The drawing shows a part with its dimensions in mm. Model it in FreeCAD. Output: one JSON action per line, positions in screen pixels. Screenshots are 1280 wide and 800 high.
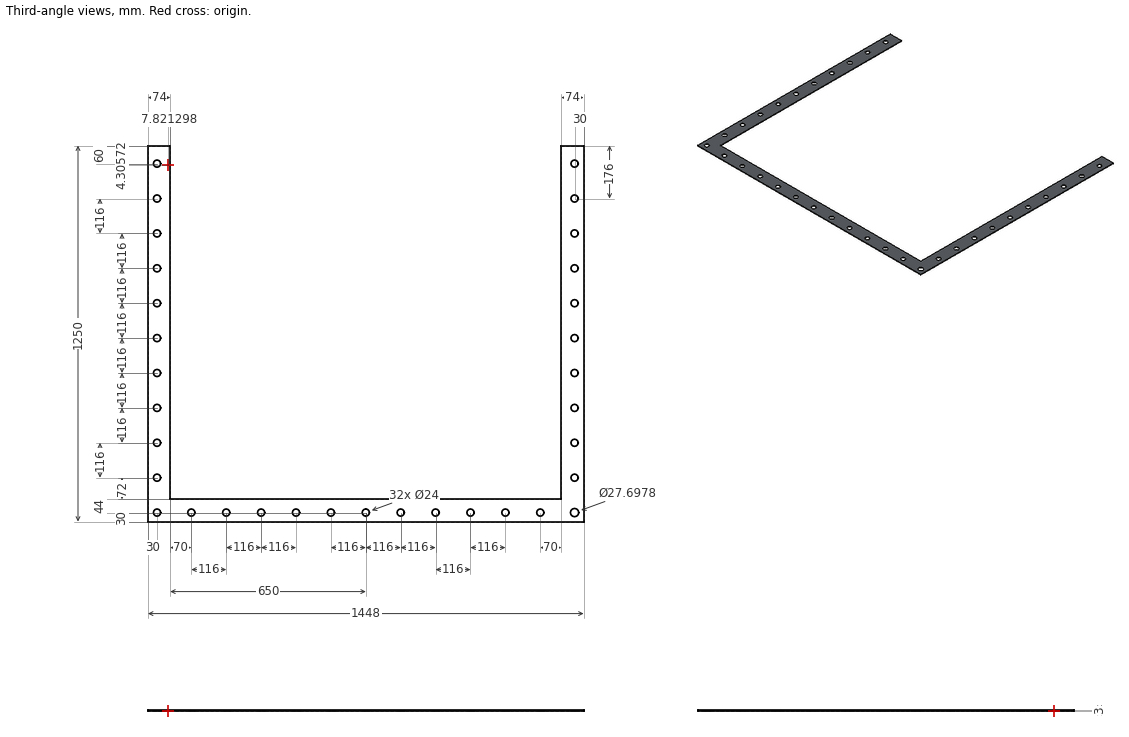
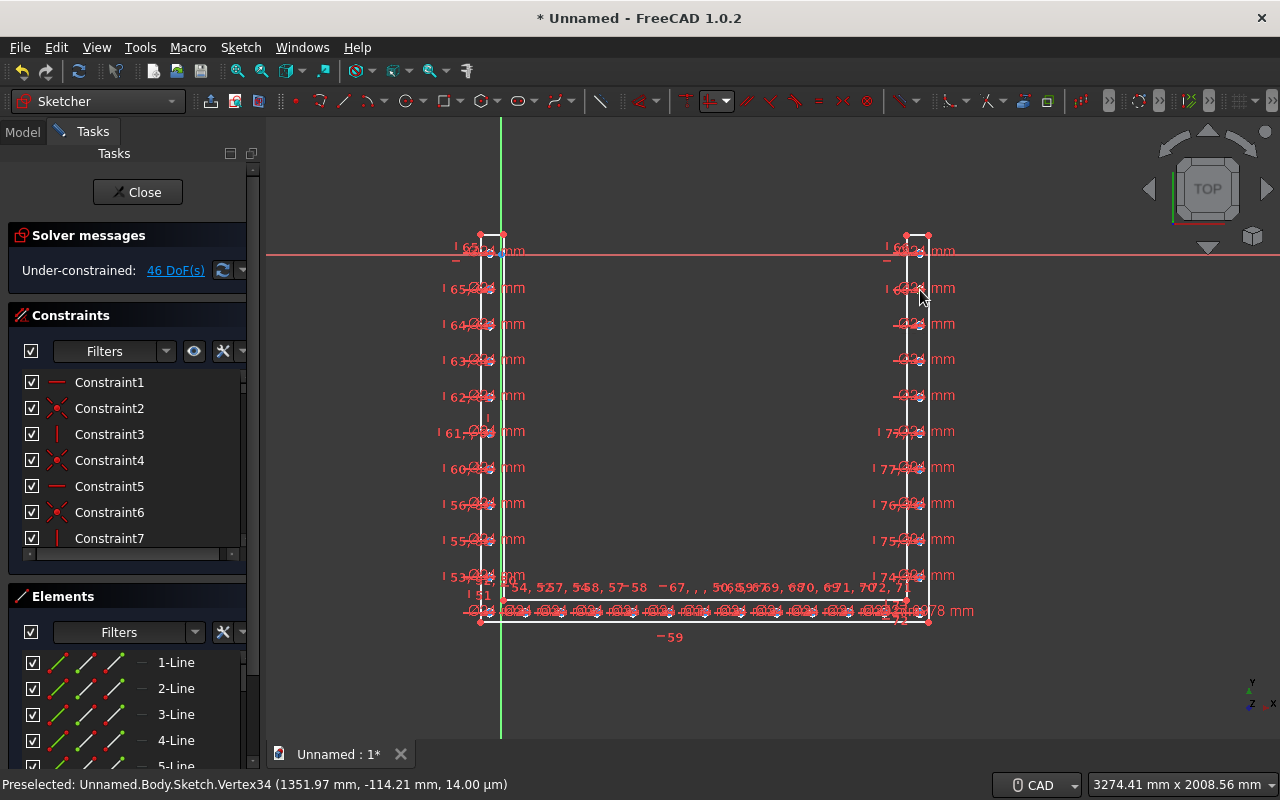
{"action": "left_click", "coordinate": [920, 433]}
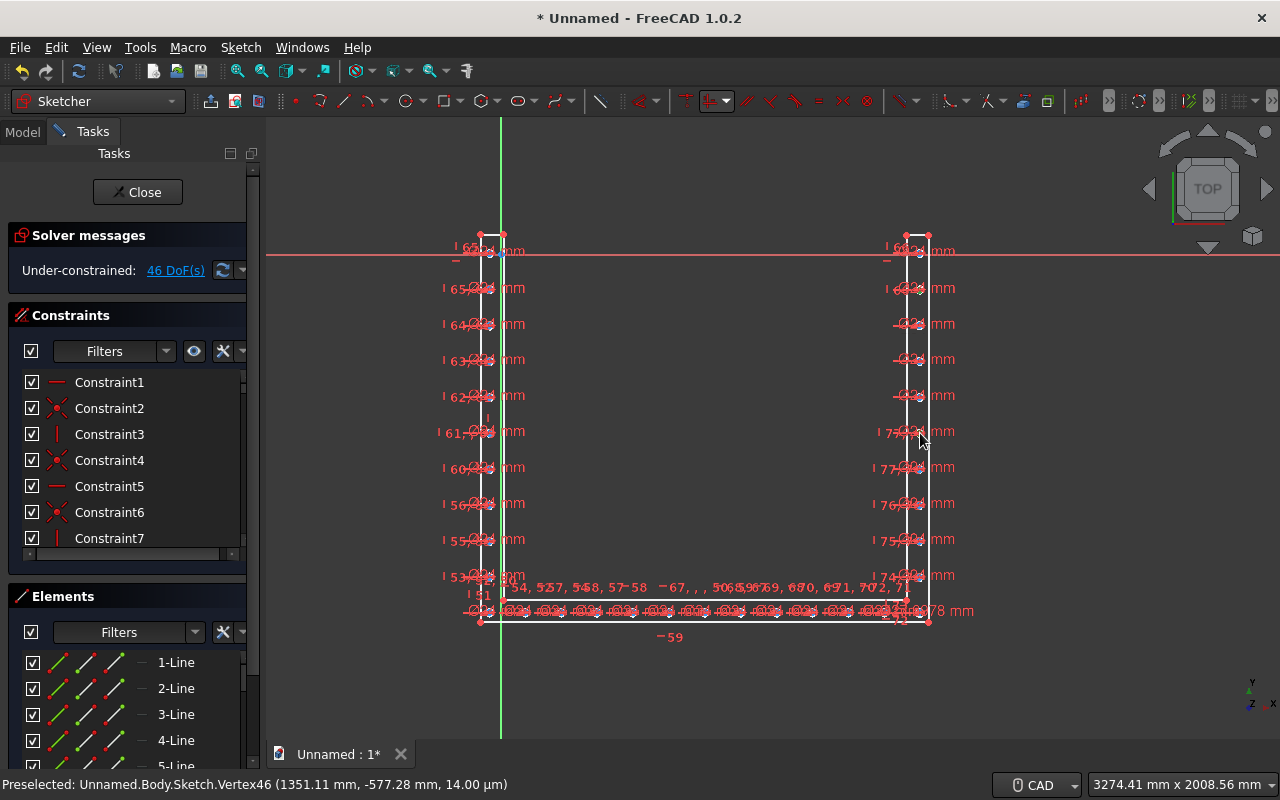
{"action": "key", "text": "v"}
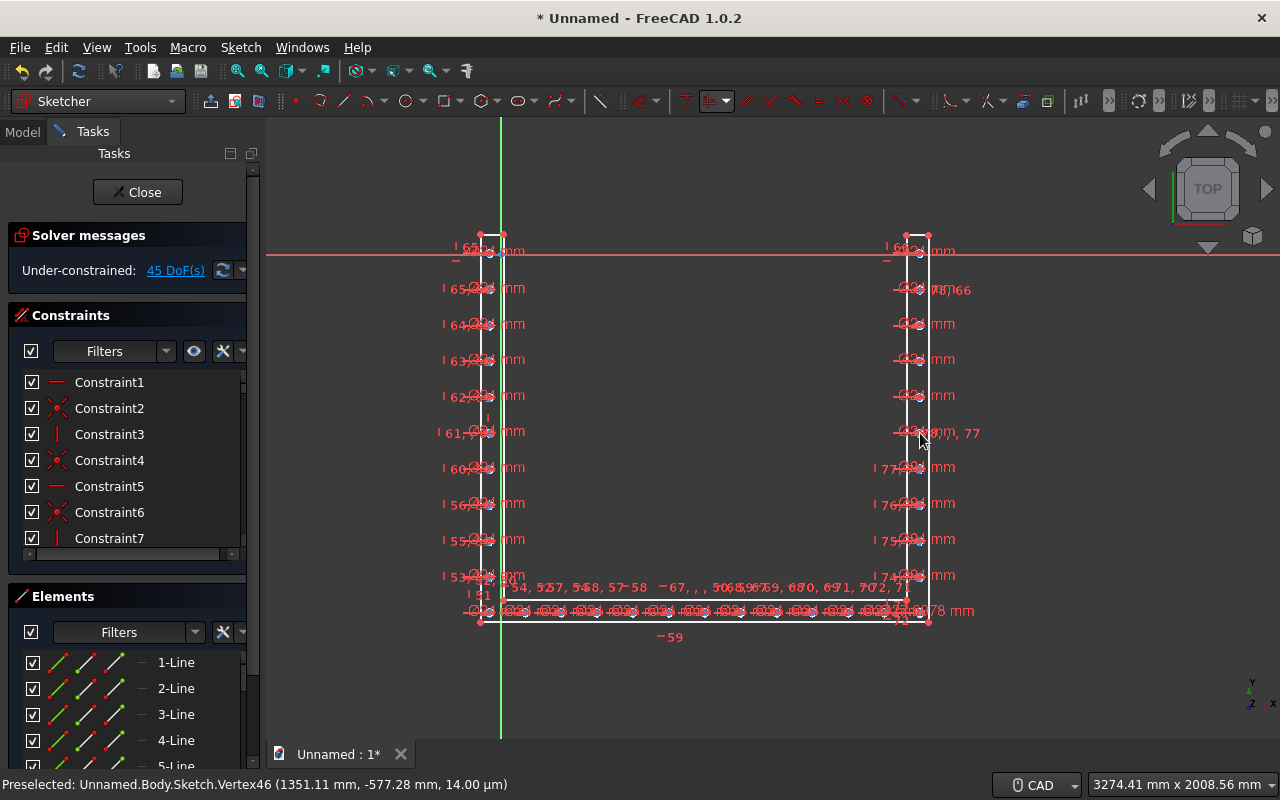
{"action": "scroll", "coordinate": [920, 433], "scroll_direction": "up", "scroll_amount": 4}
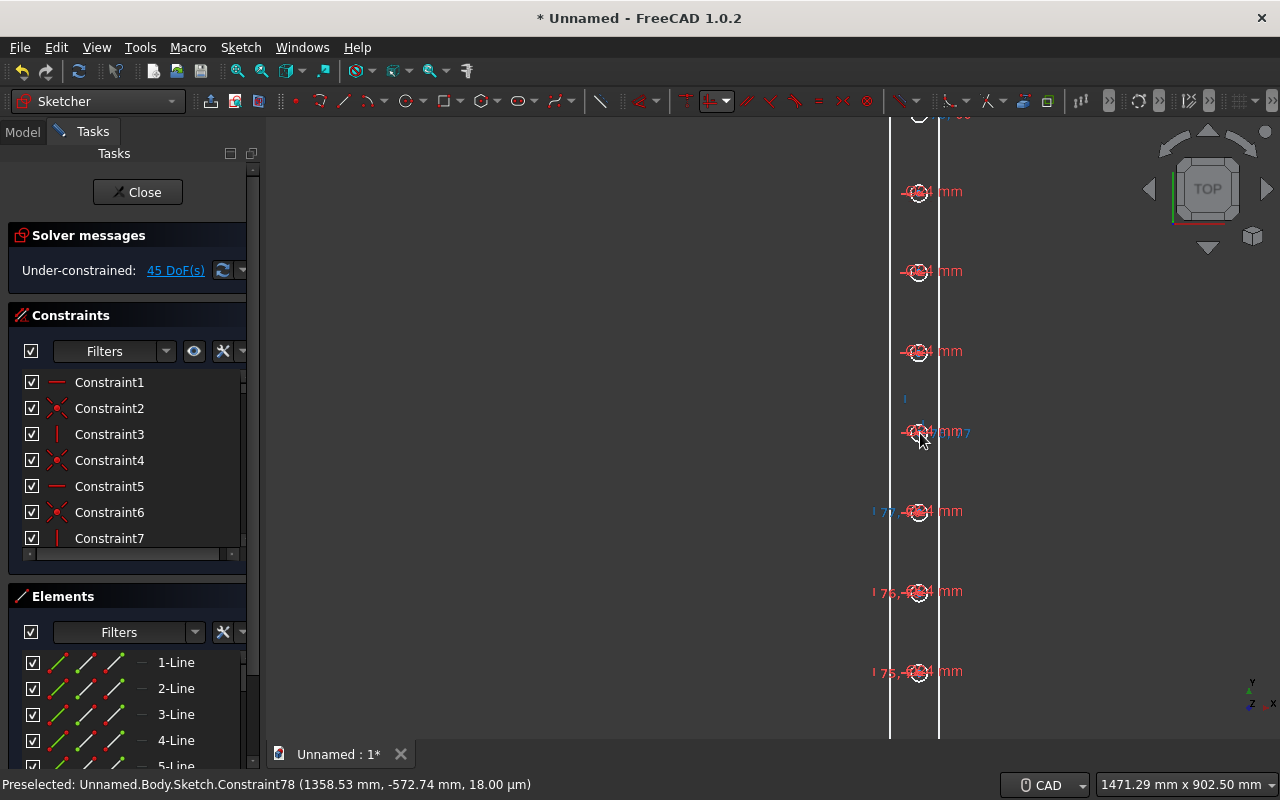
{"action": "left_click", "coordinate": [917, 435]}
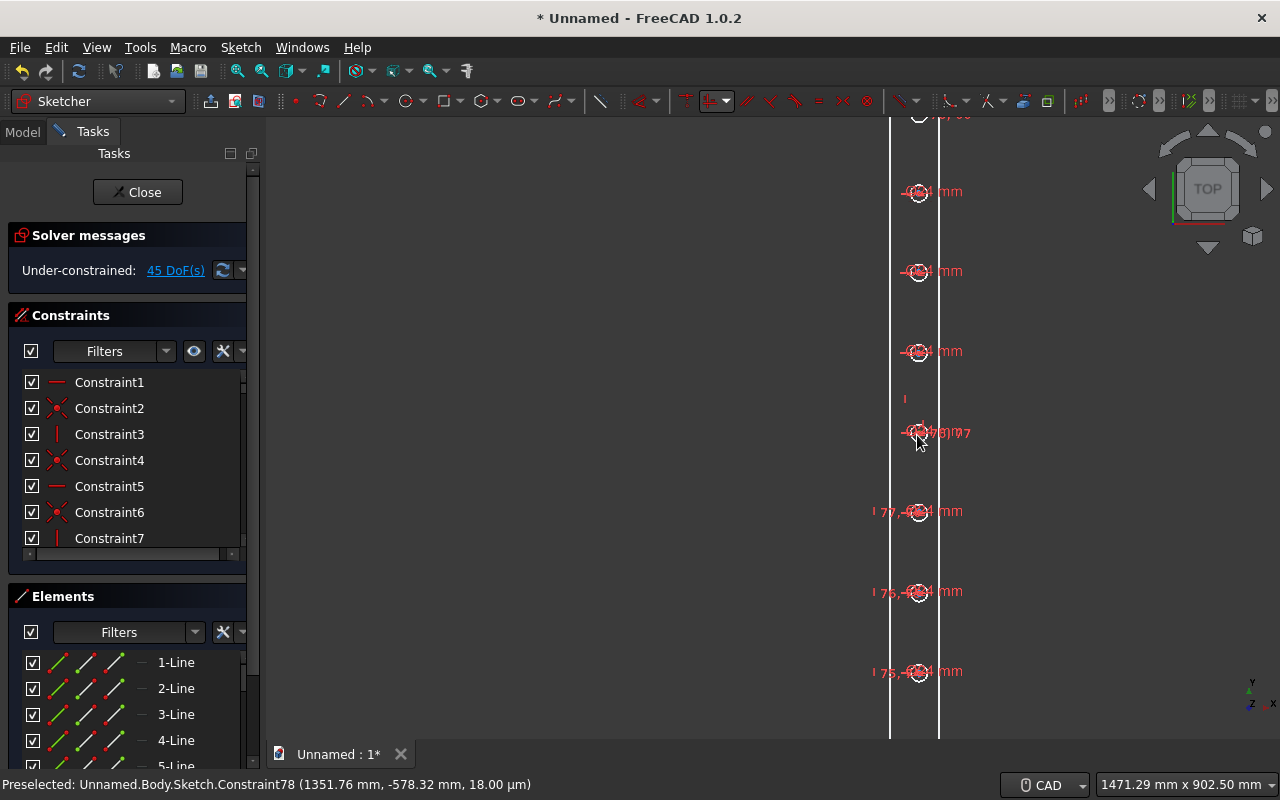
{"action": "left_click", "coordinate": [919, 353]}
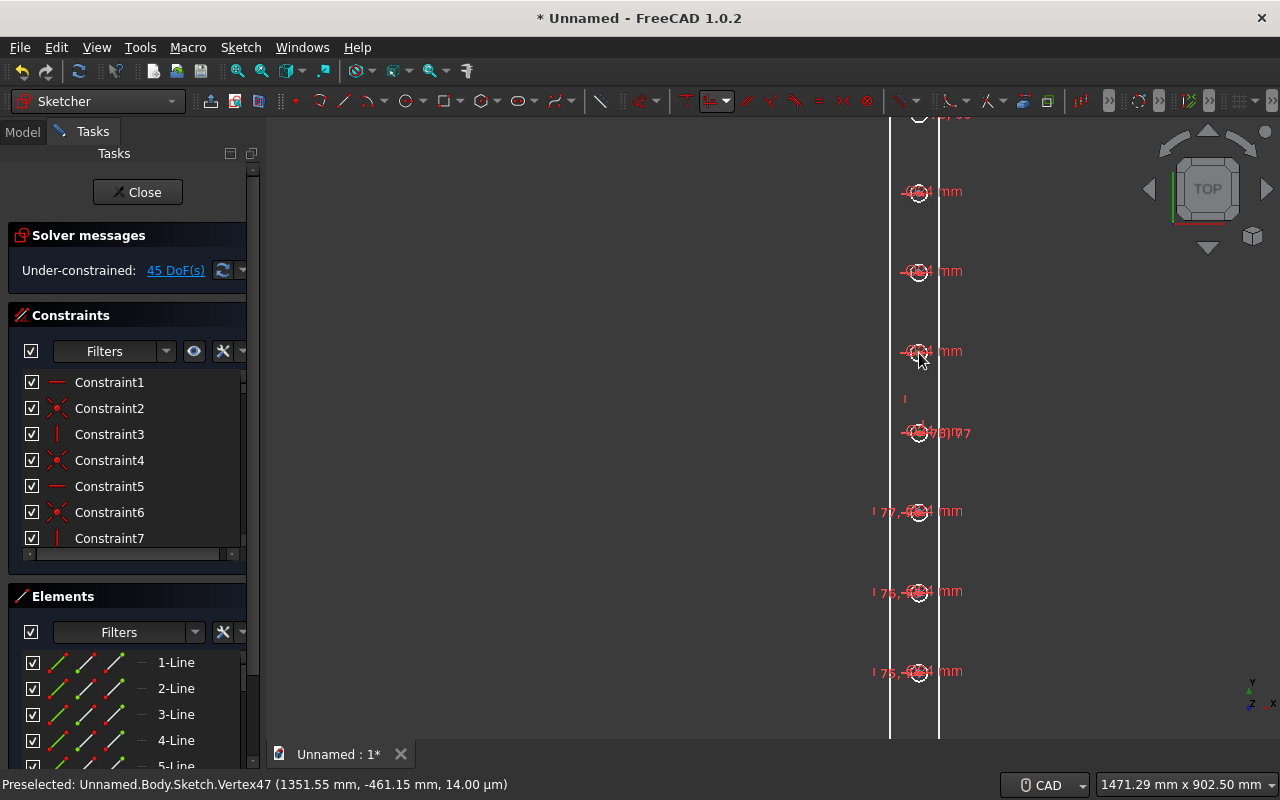
{"action": "left_click", "coordinate": [728, 102]}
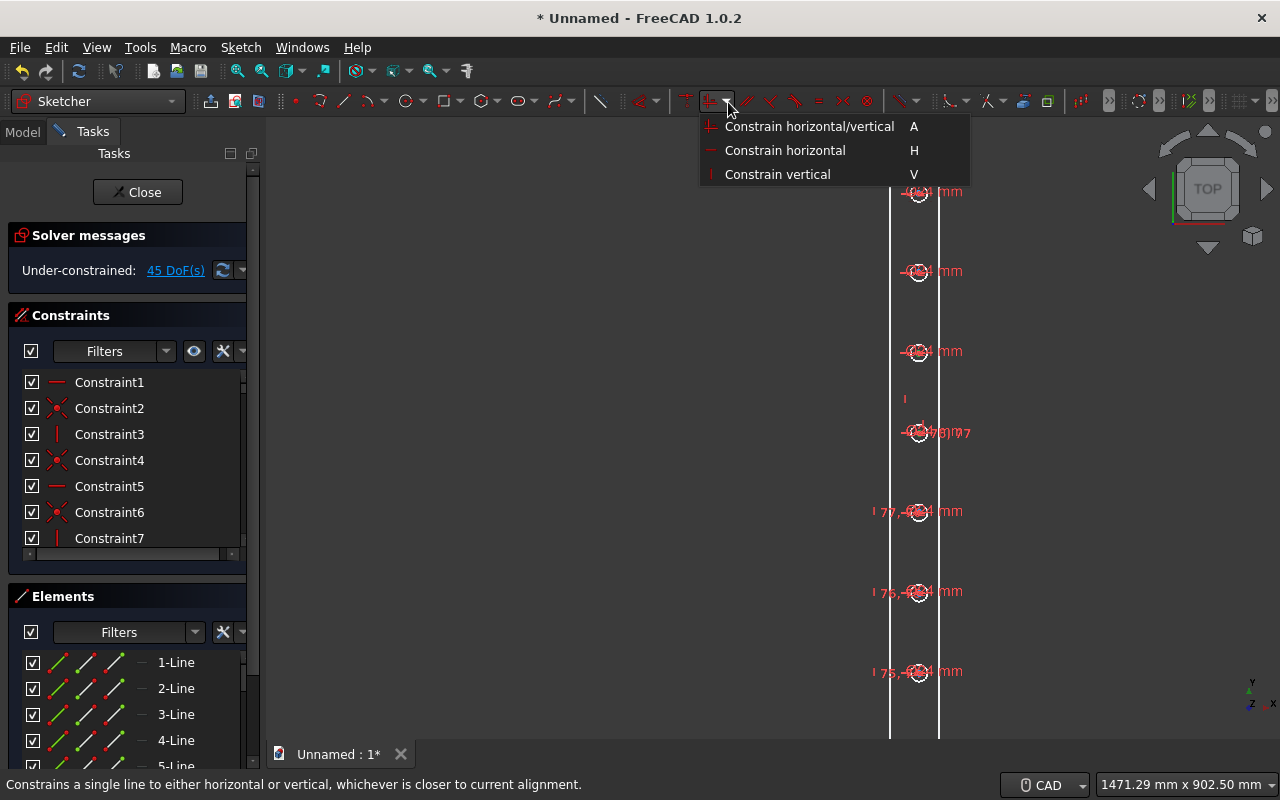
{"action": "left_click", "coordinate": [835, 174]}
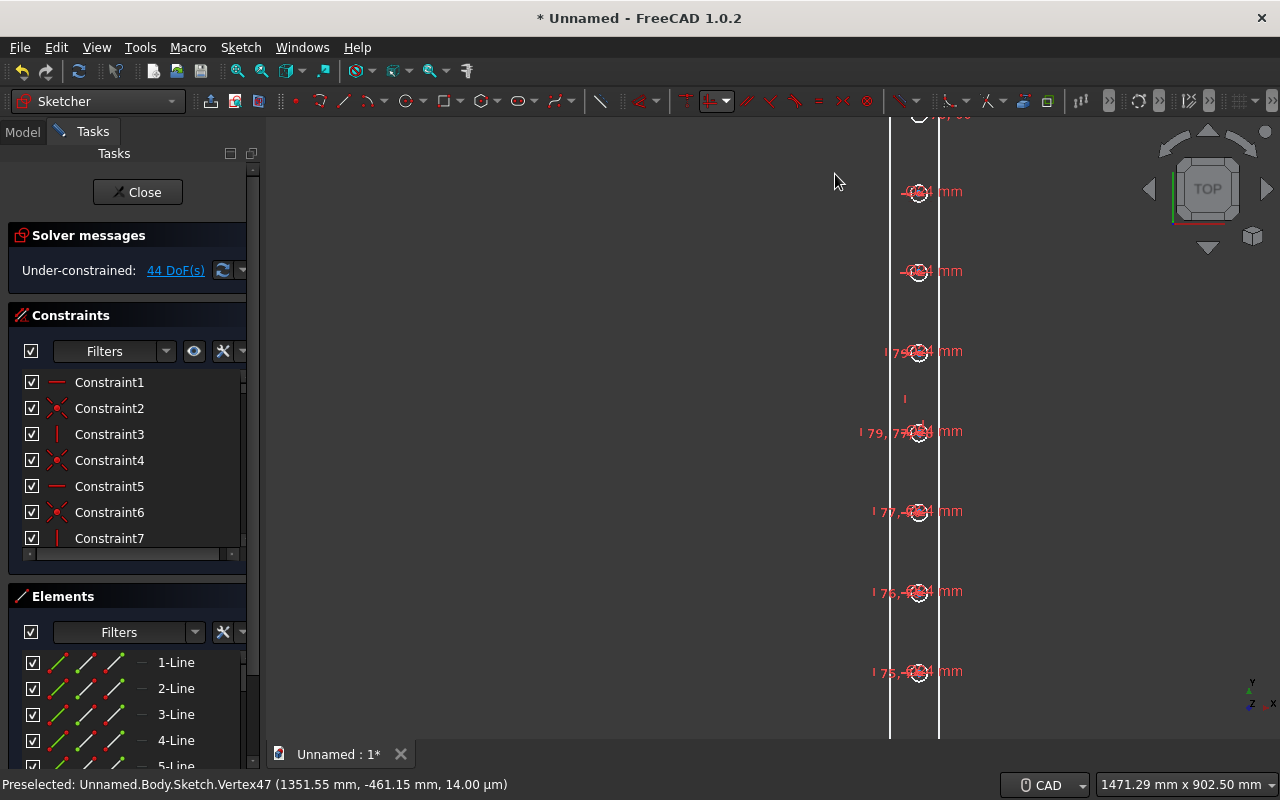
{"action": "left_click", "coordinate": [919, 353]}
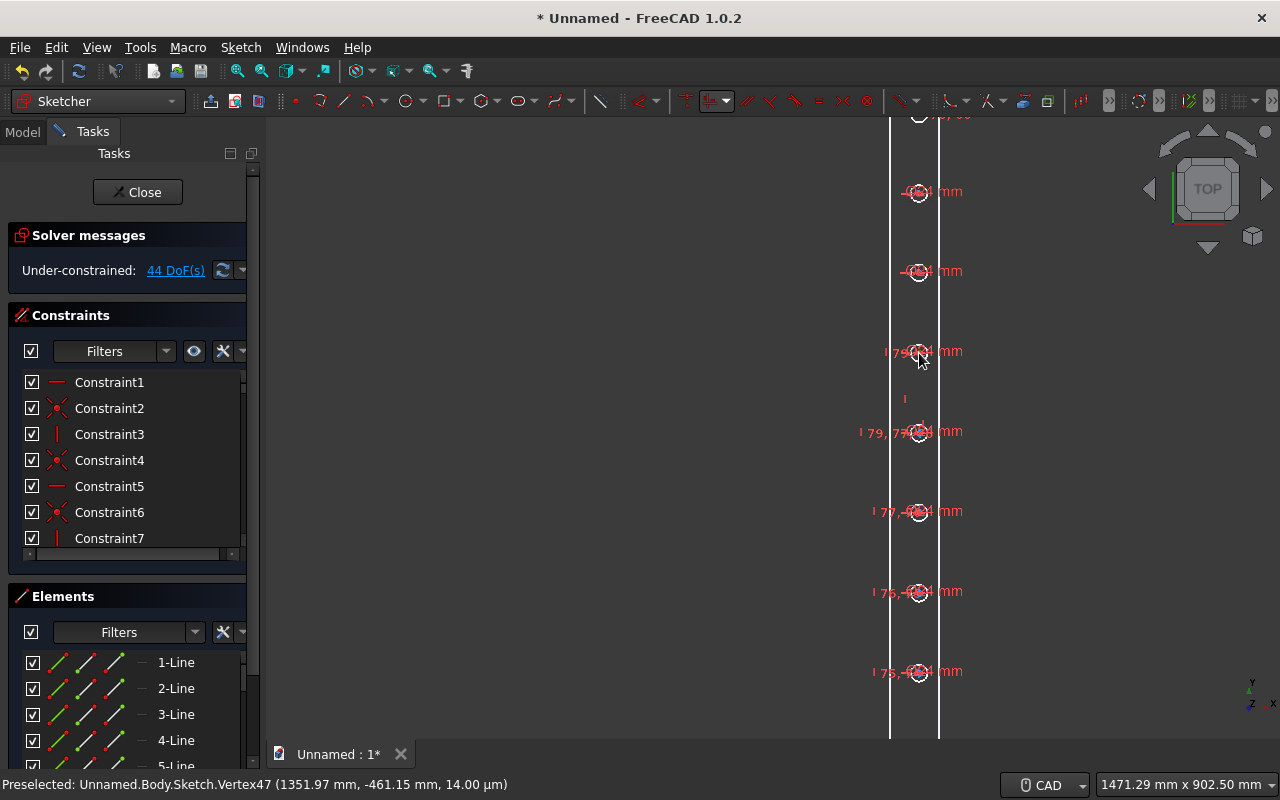
{"action": "left_click", "coordinate": [919, 273]}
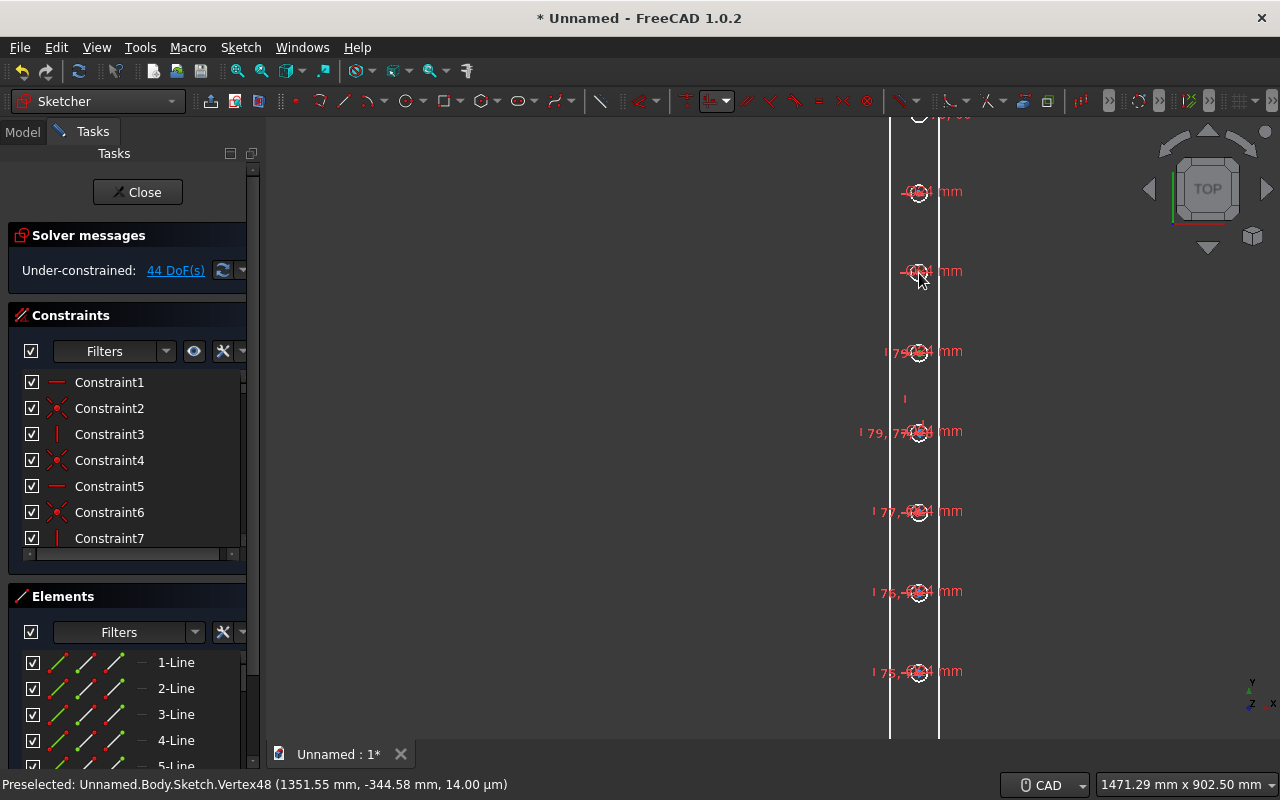
{"action": "left_click", "coordinate": [728, 102]}